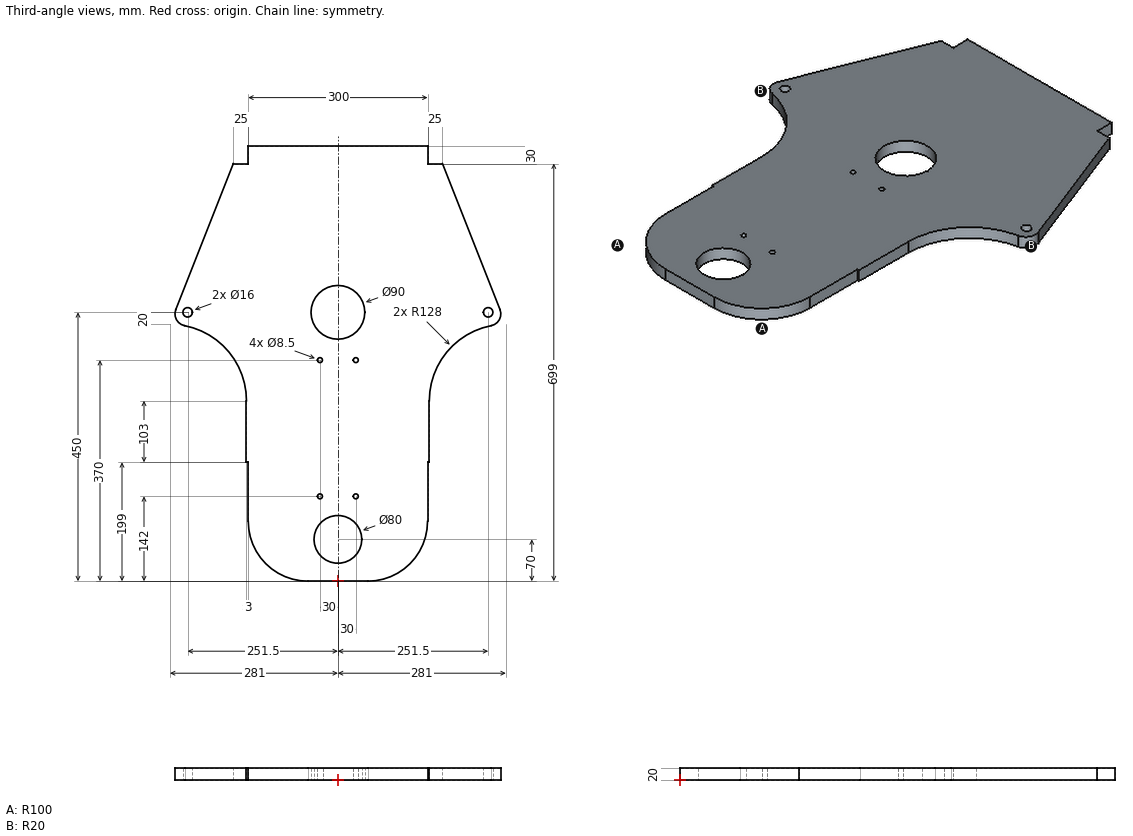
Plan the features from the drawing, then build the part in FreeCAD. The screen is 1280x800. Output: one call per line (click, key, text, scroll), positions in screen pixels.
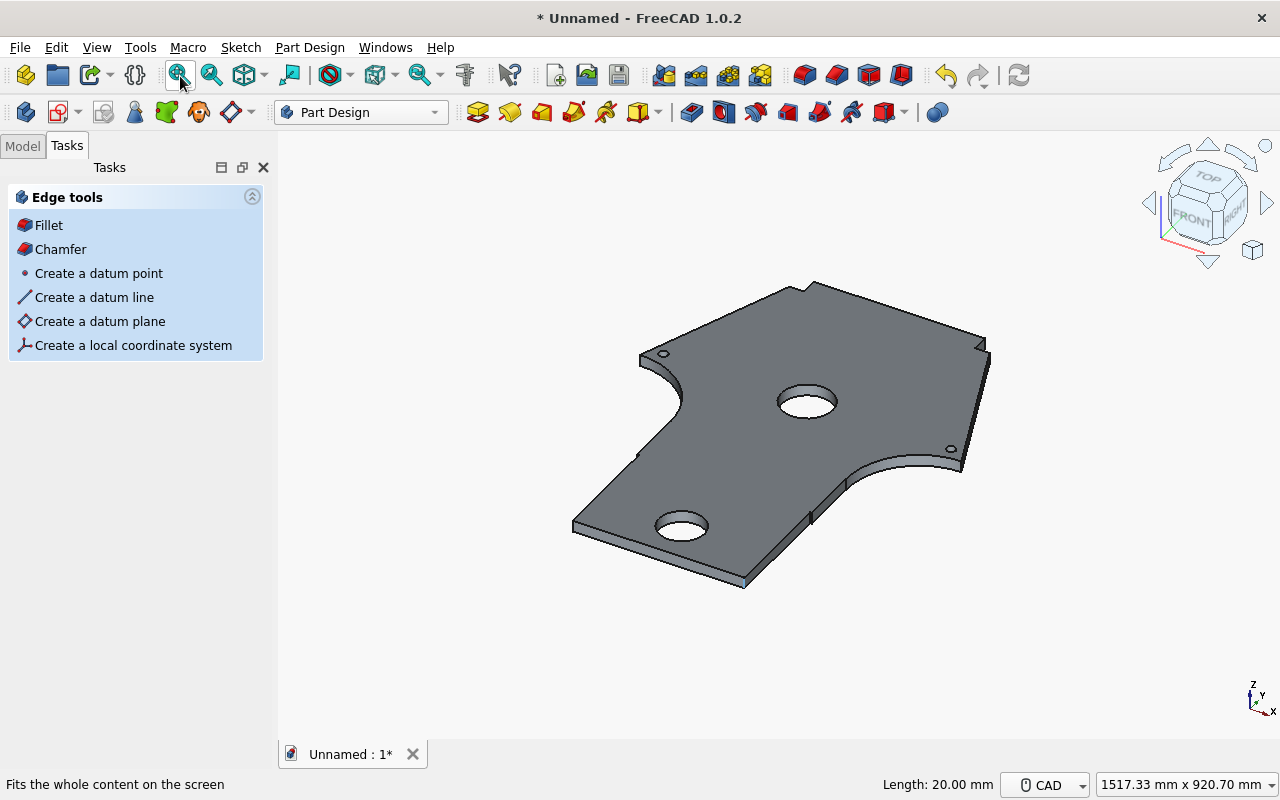
key(0)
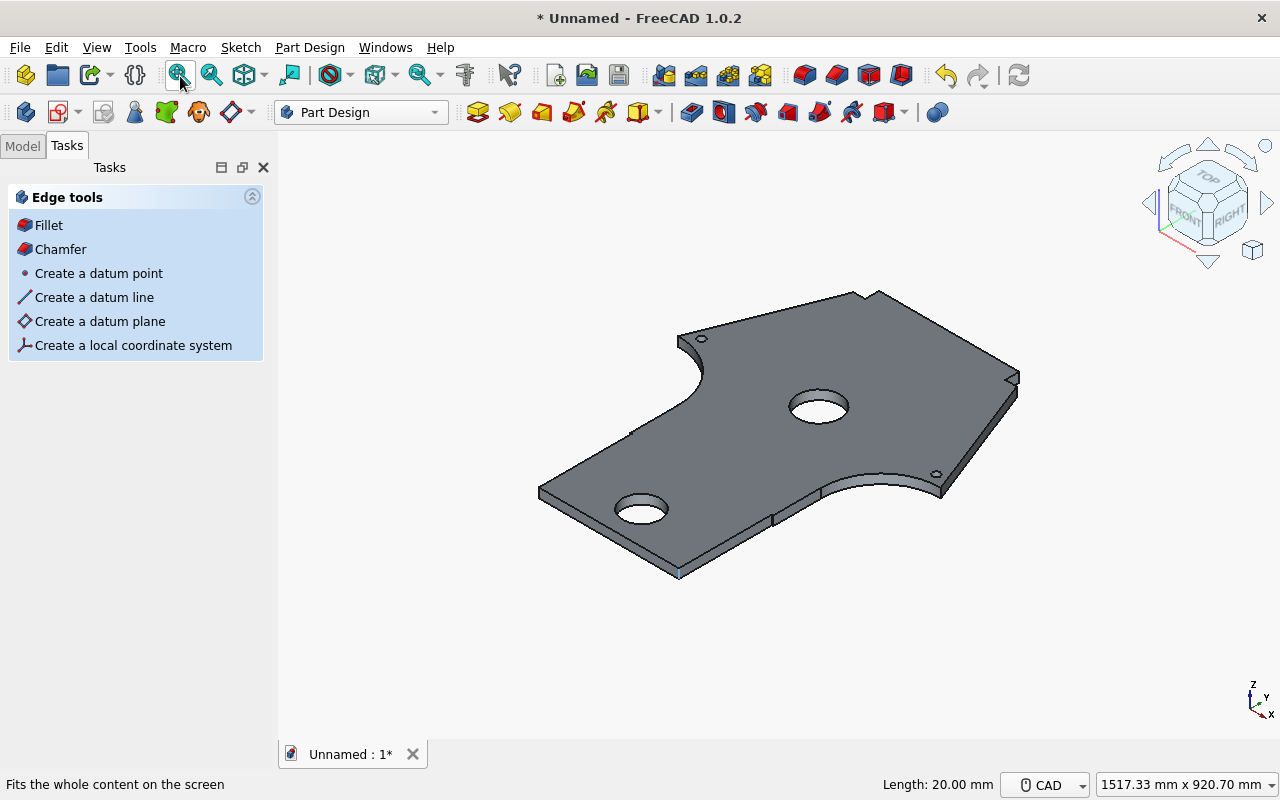
scroll(539, 492, up, 6)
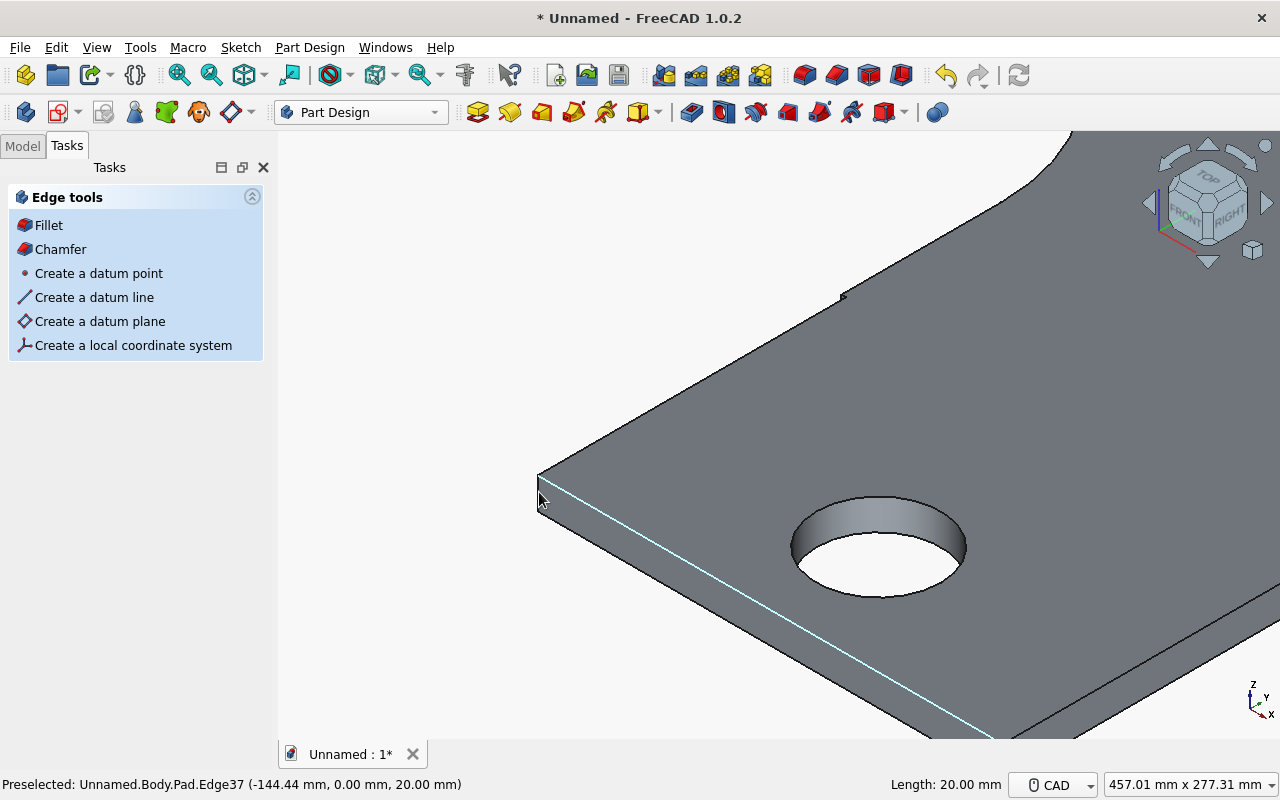
click(180, 76)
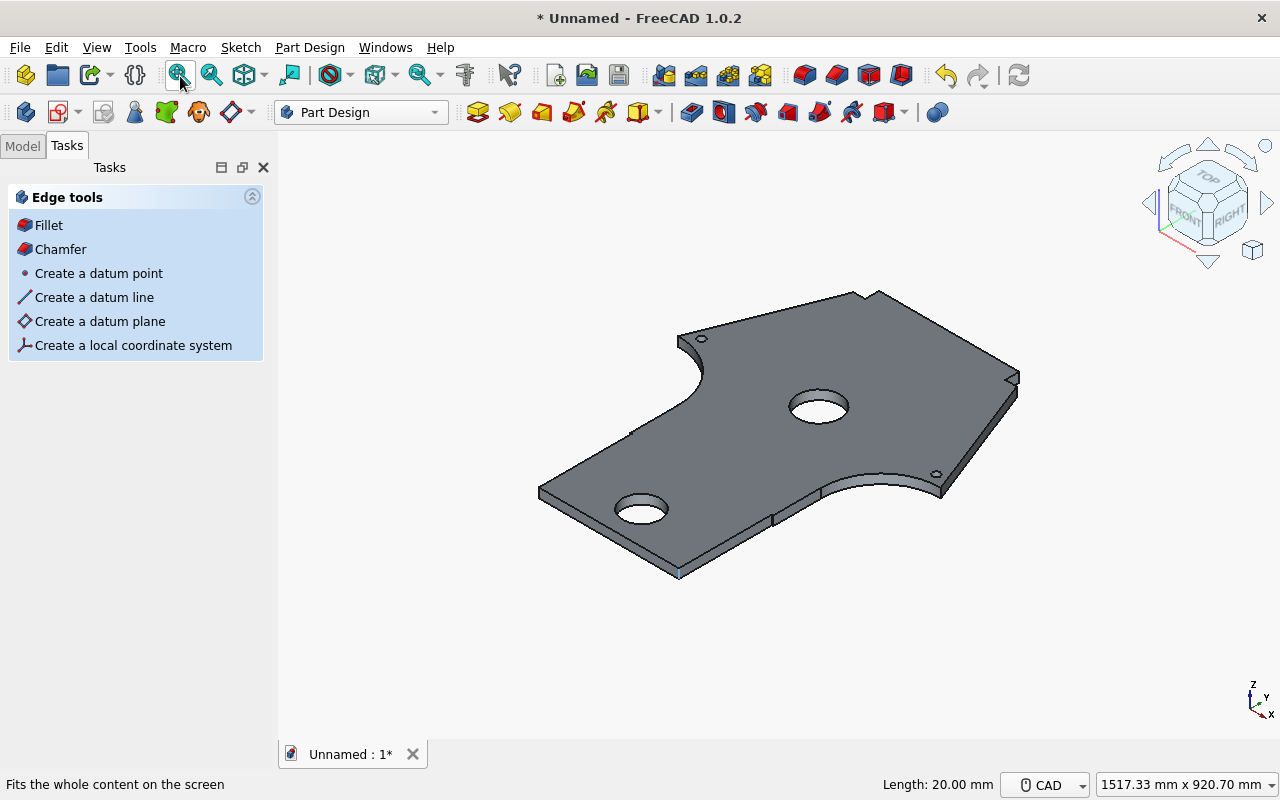
key(2)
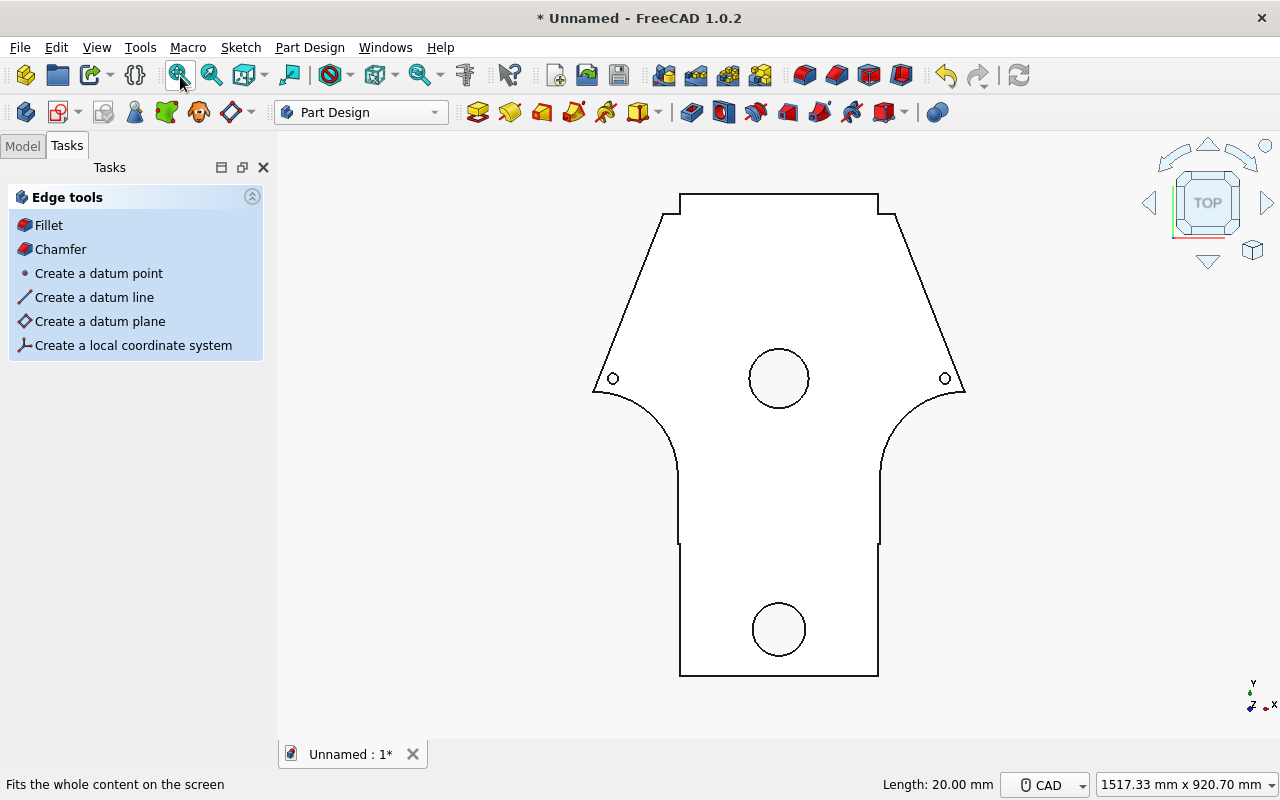
scroll(680, 675, up, 6)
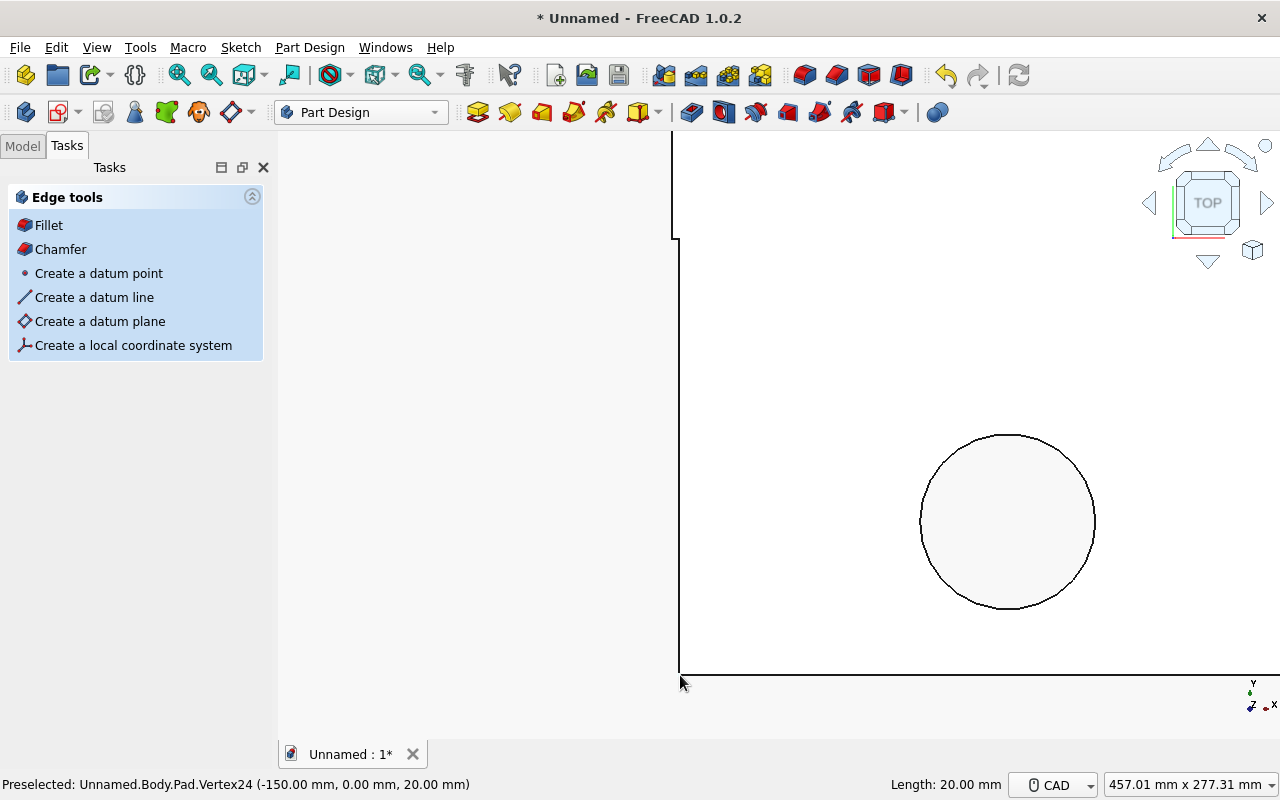
key(v)
key(f)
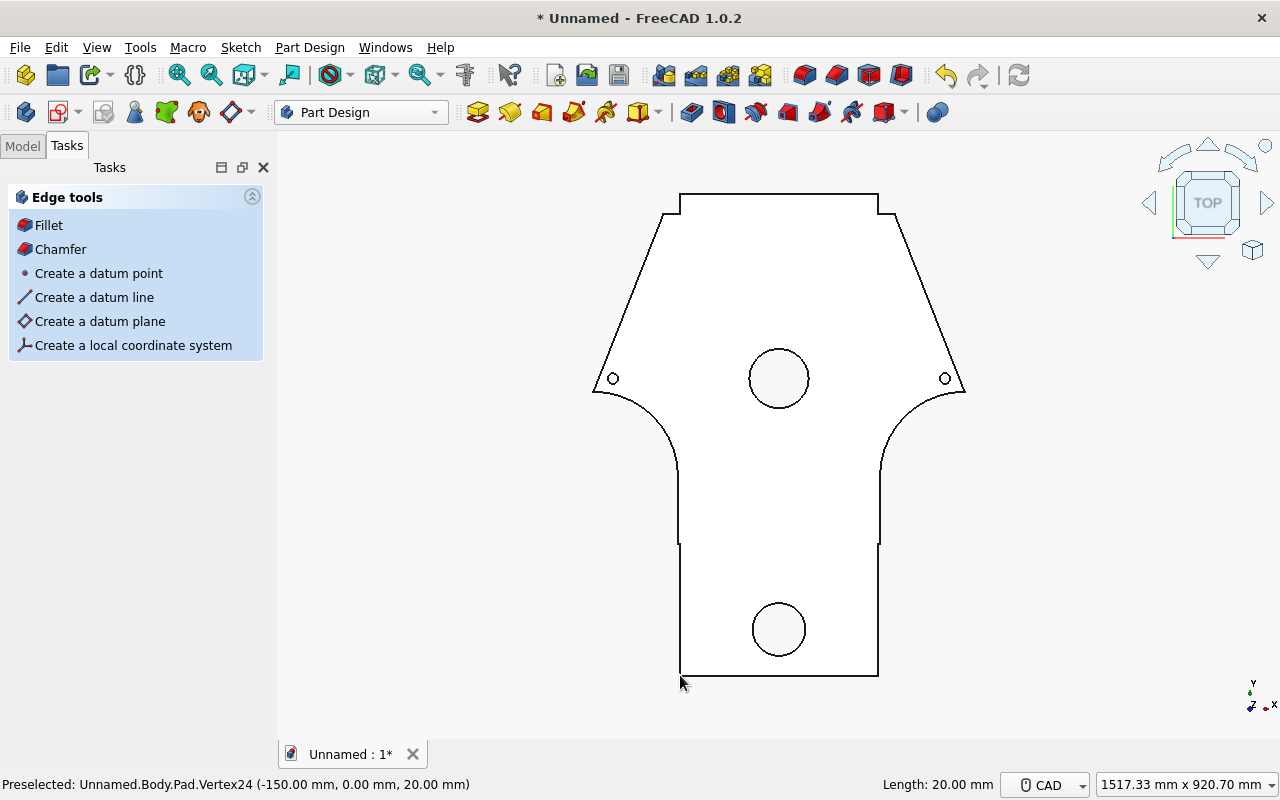
key(1)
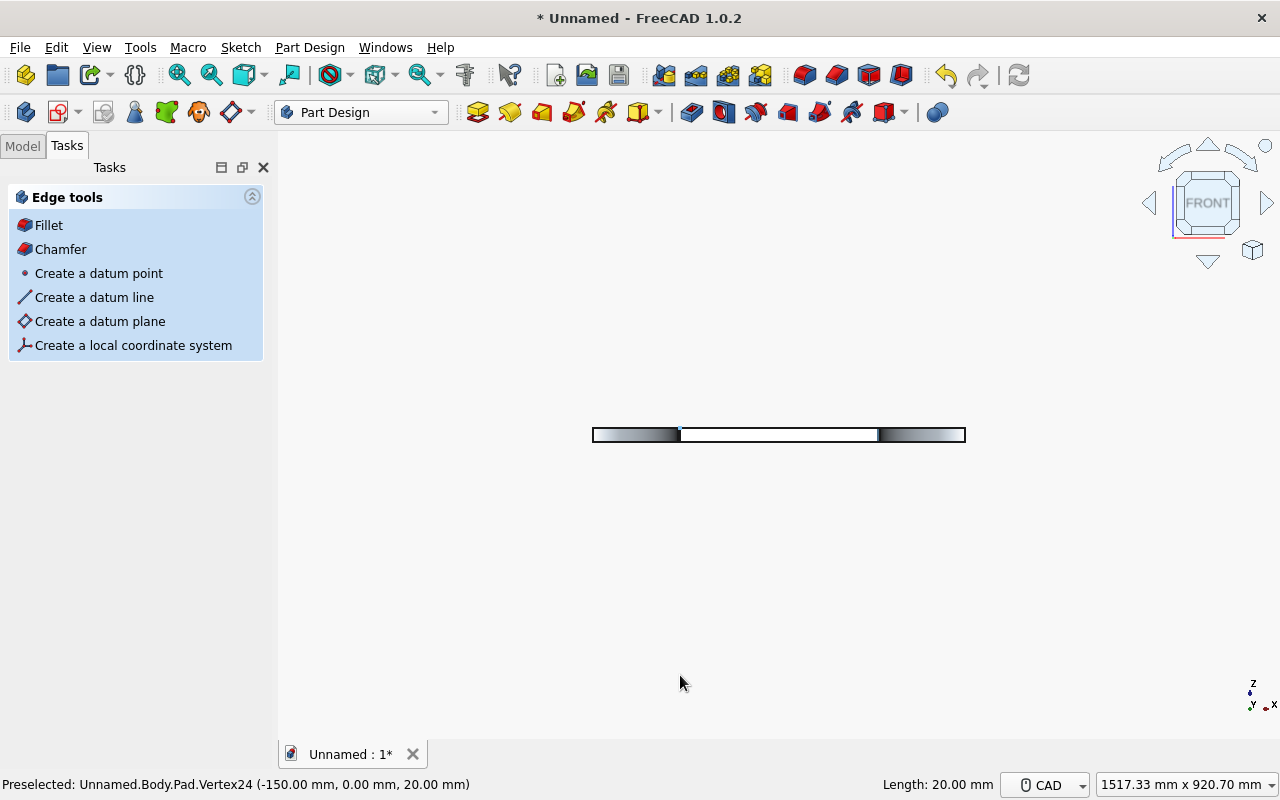
click(180, 76)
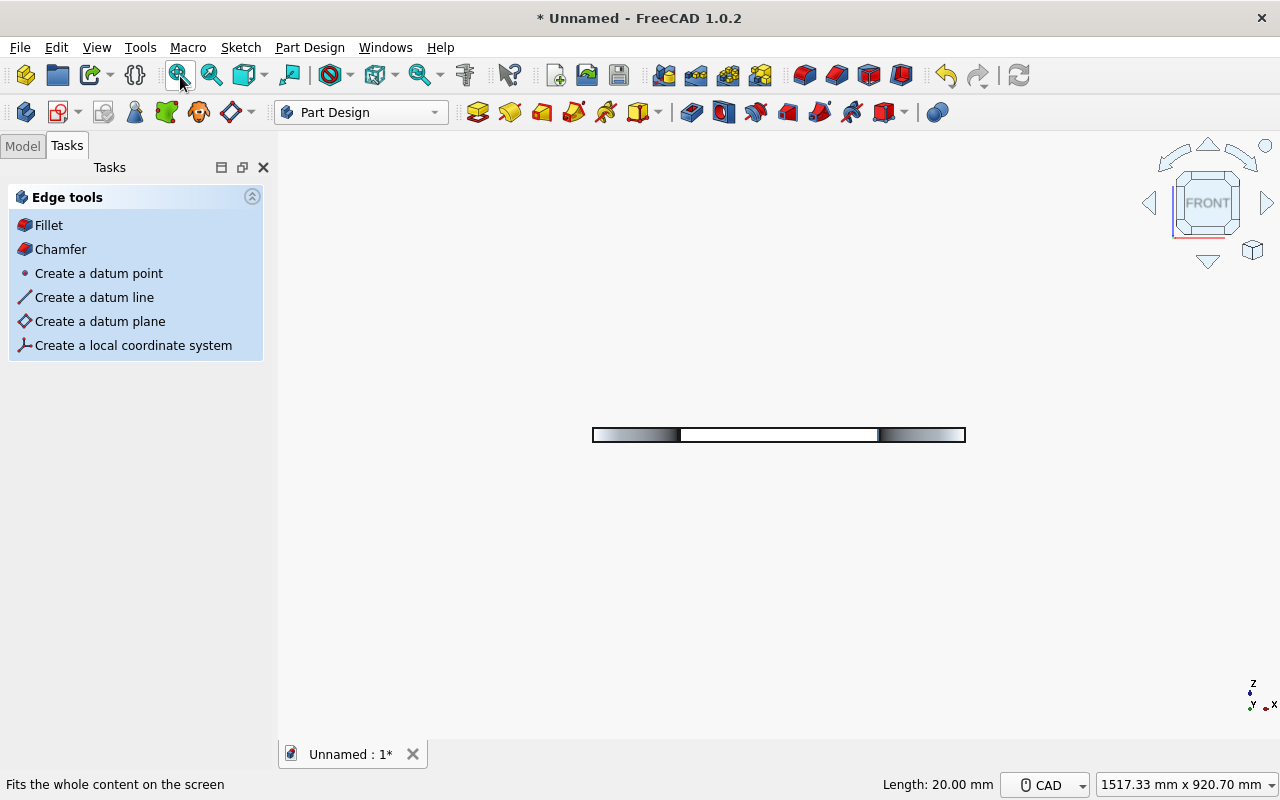
click(680, 434, ctrl)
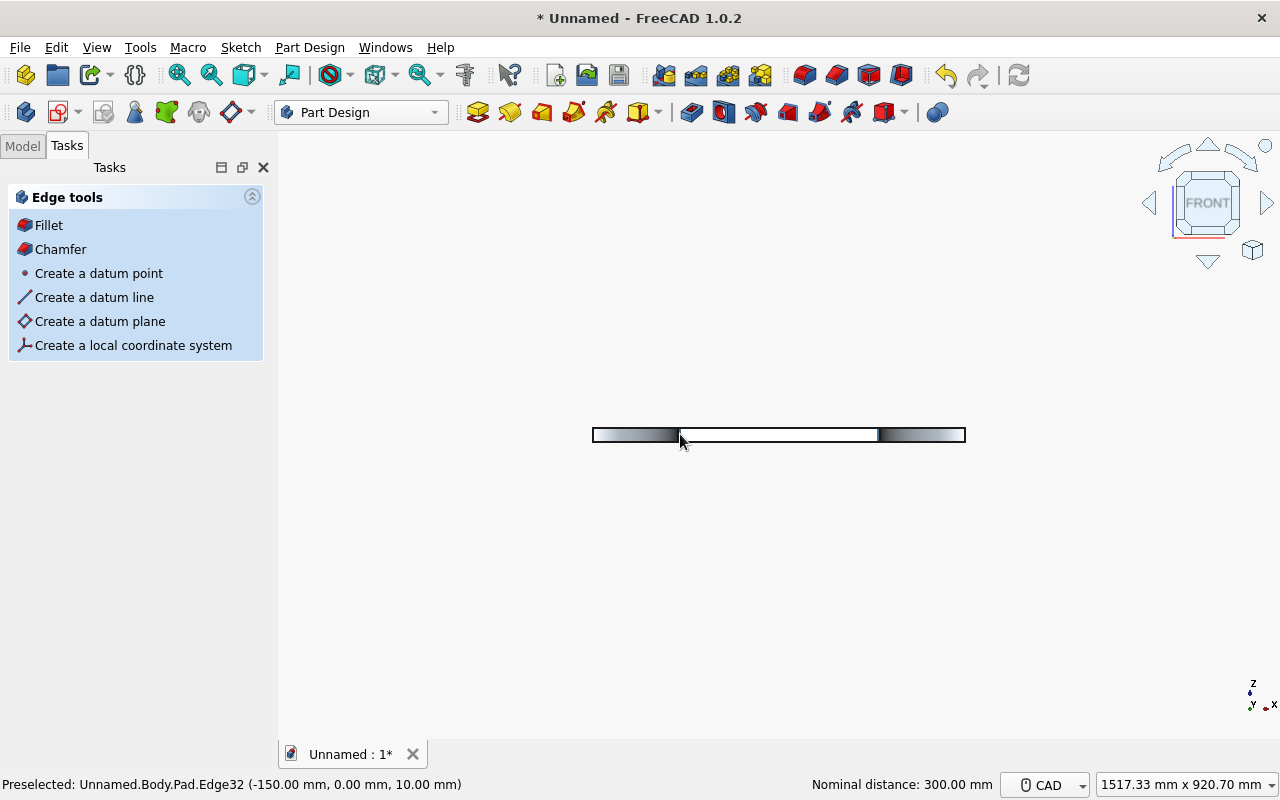
click(806, 76)